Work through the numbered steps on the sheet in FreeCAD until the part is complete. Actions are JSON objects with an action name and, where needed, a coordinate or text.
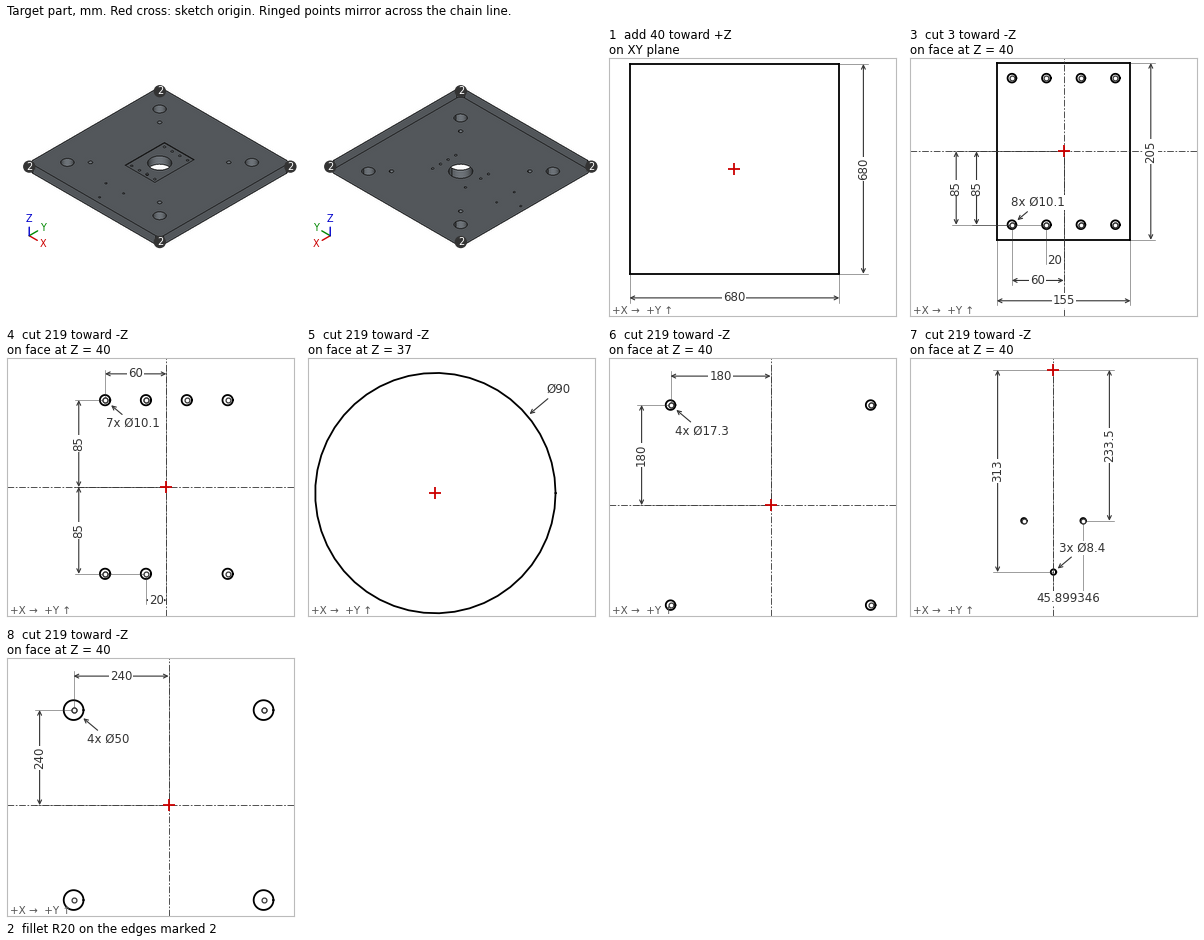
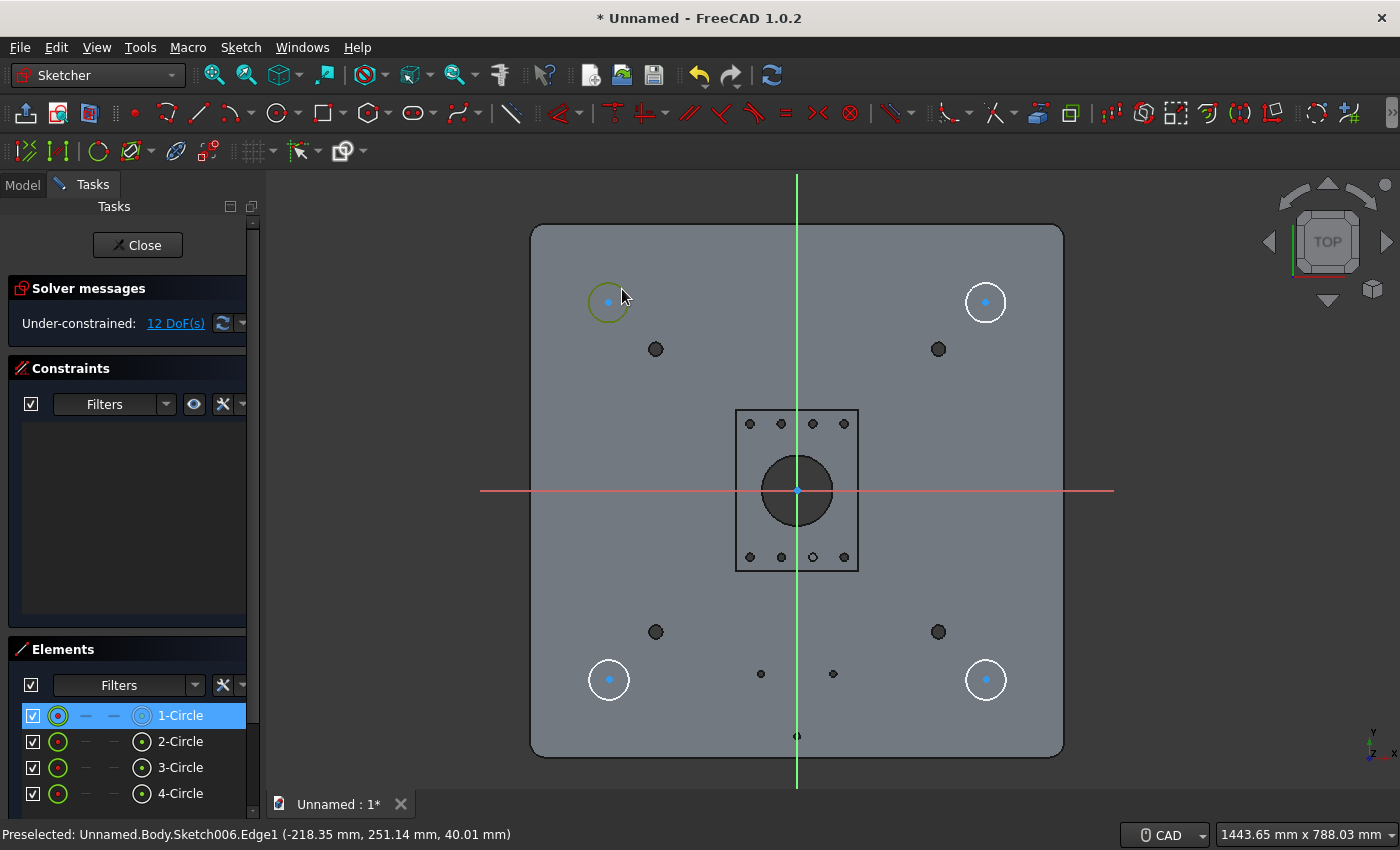
{"action": "left_click", "coordinate": [1000, 289]}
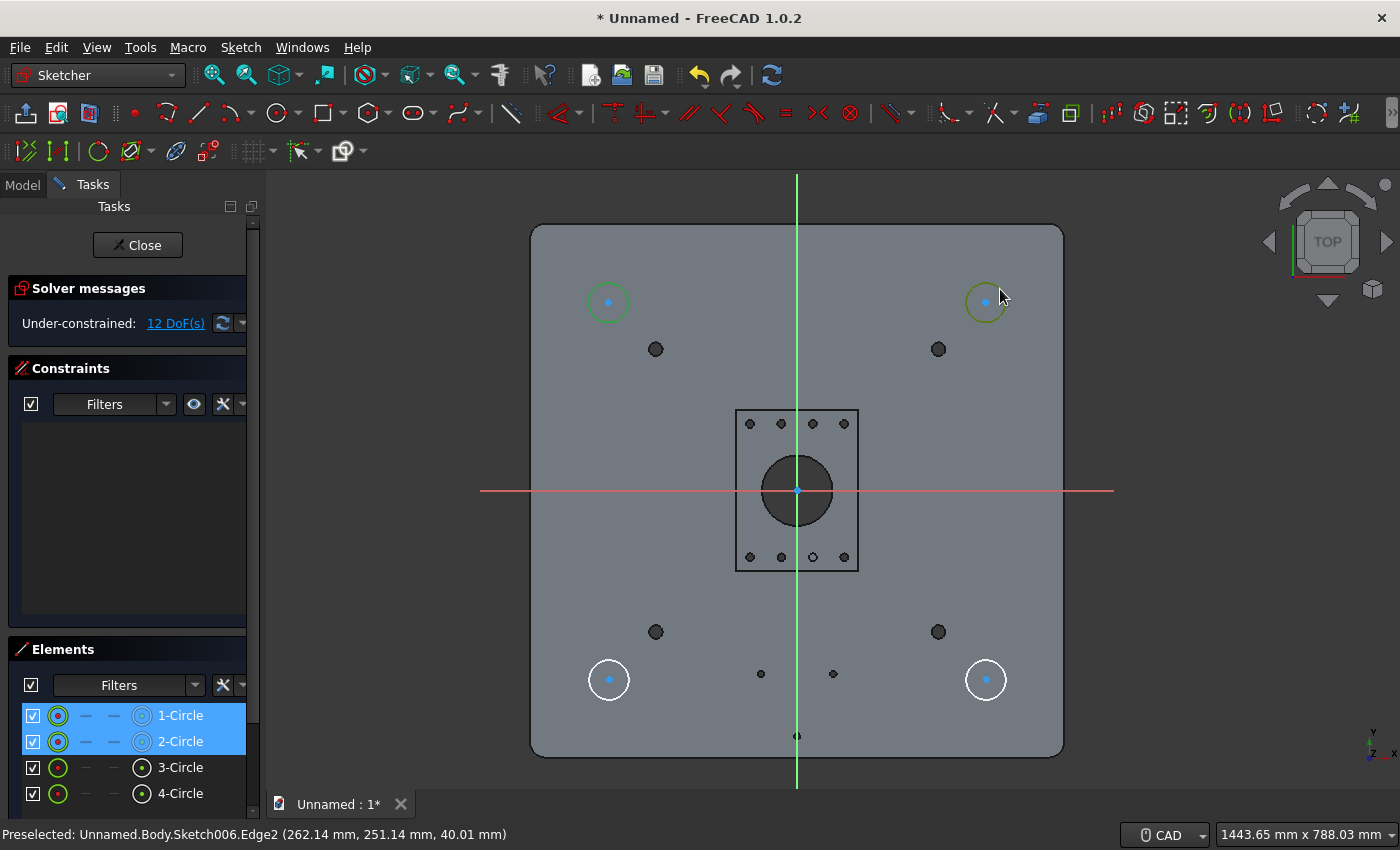
{"action": "left_click", "coordinate": [1000, 666]}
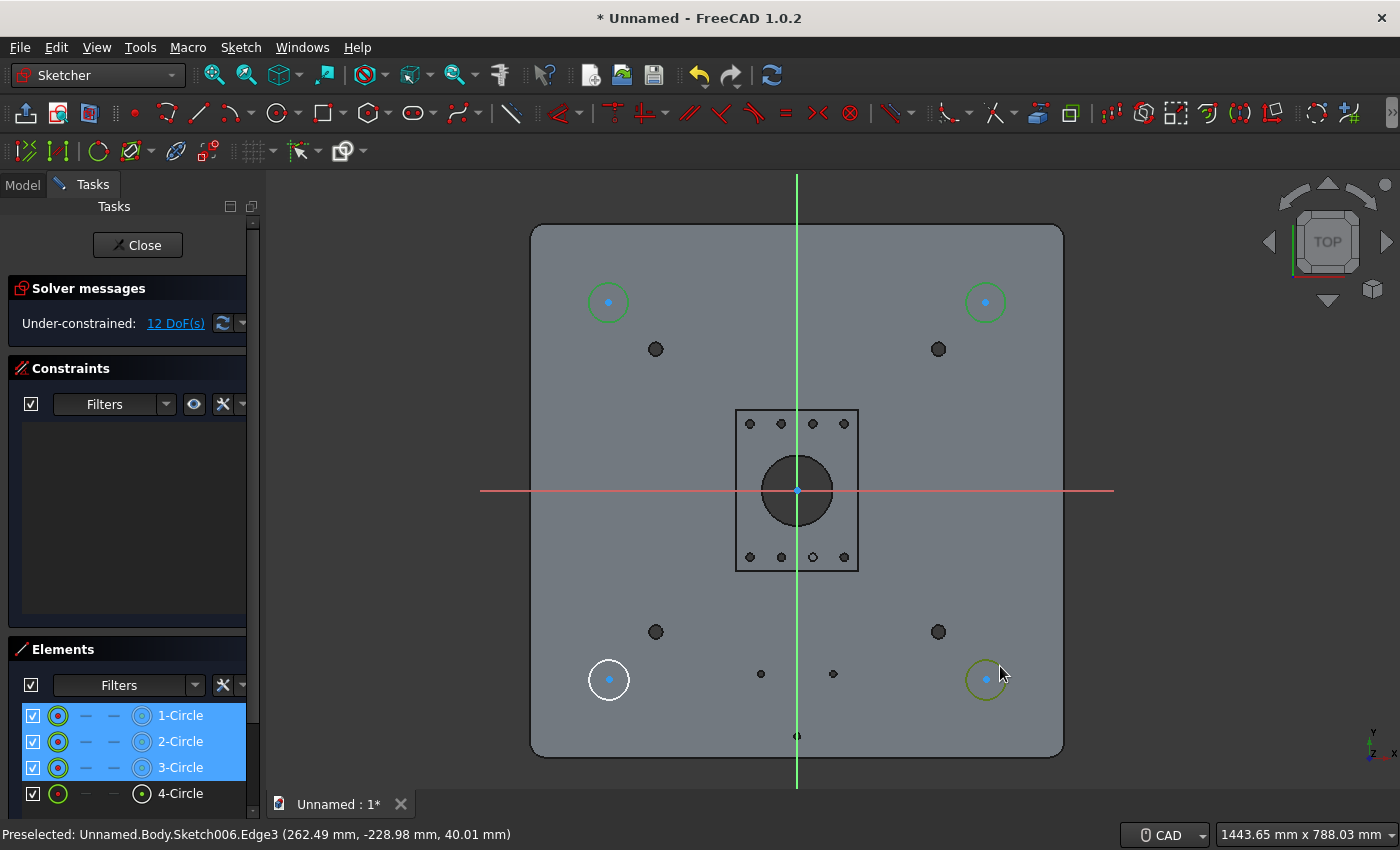
{"action": "left_click", "coordinate": [623, 666]}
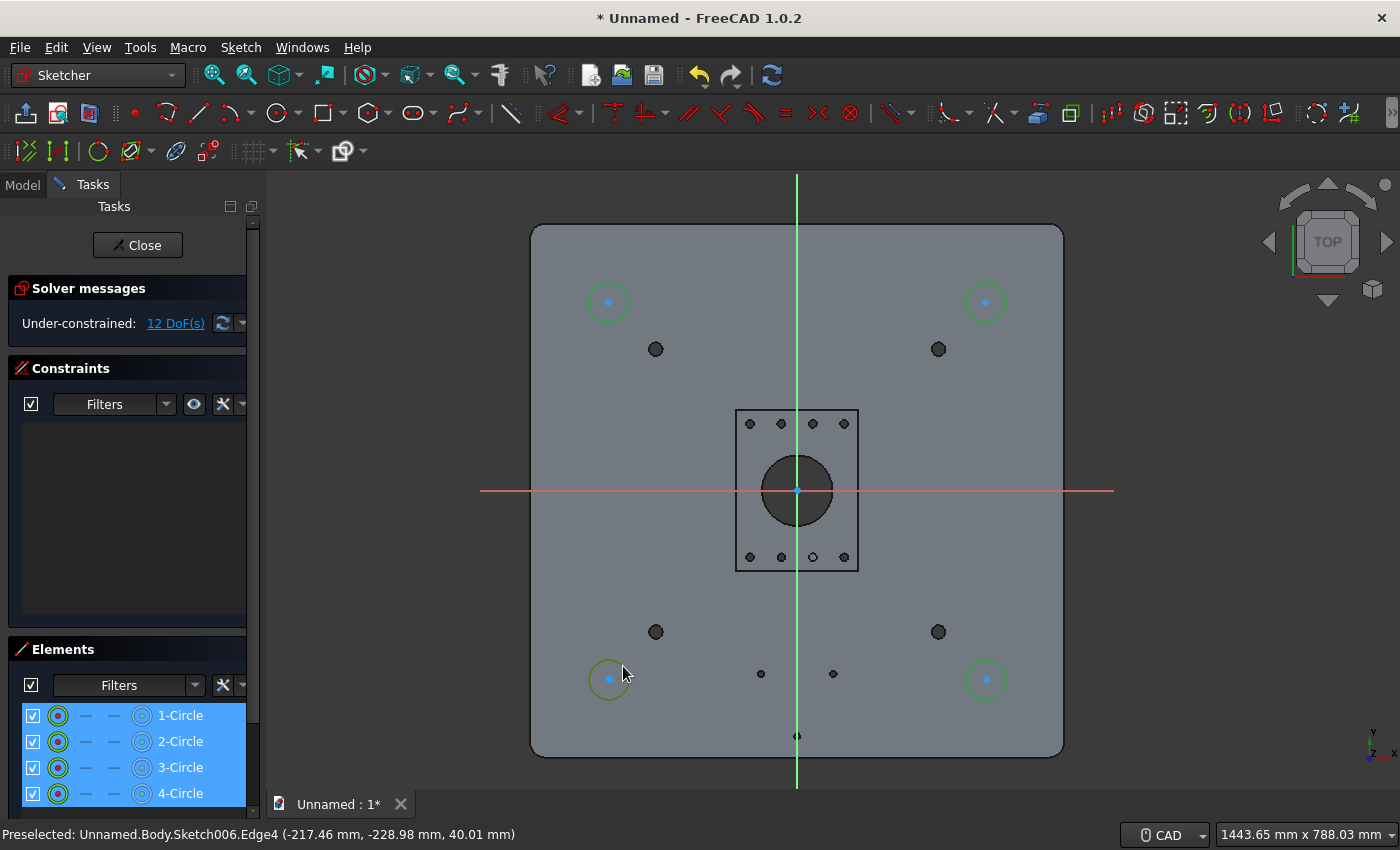
{"action": "left_click", "coordinate": [786, 114]}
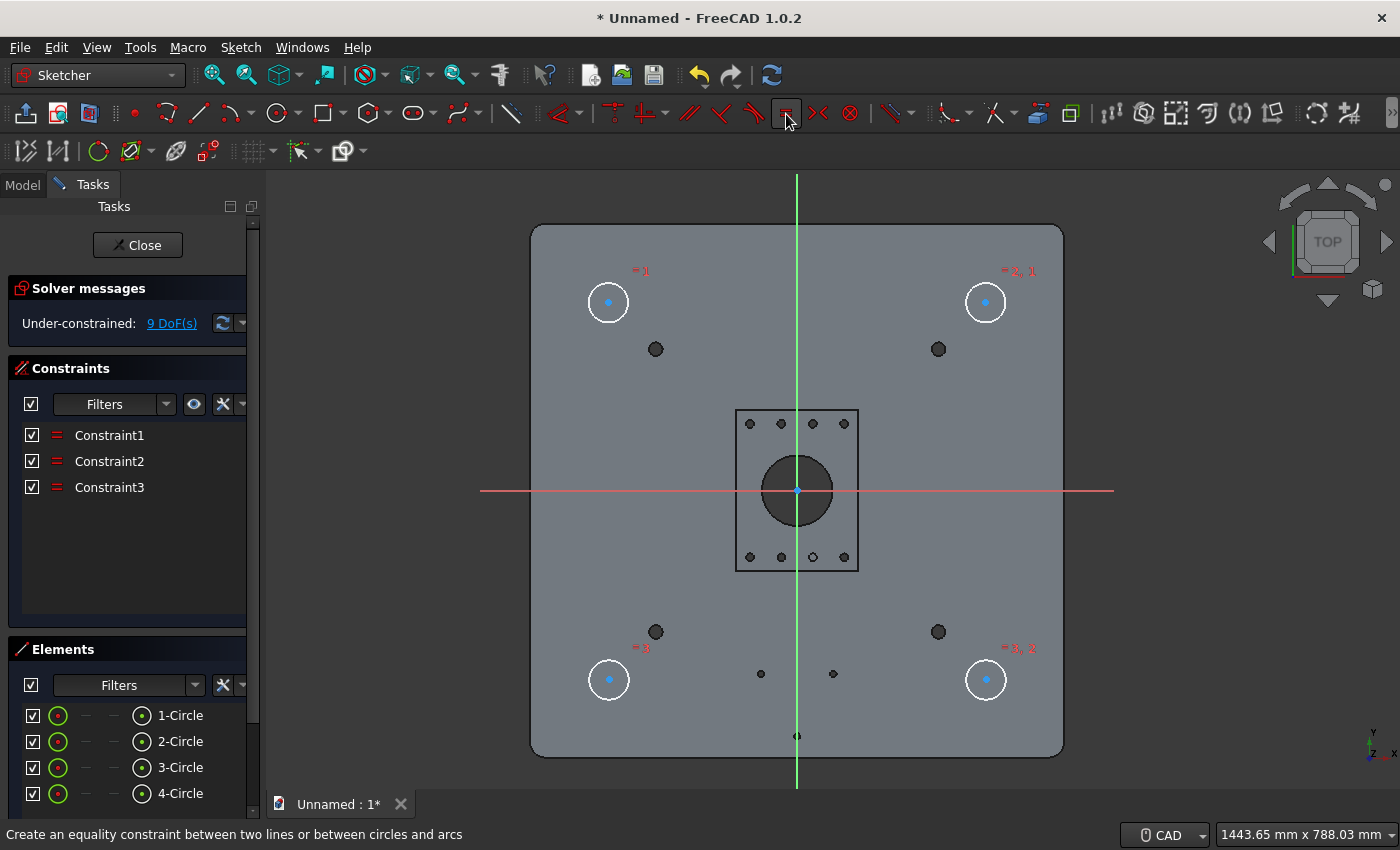
{"action": "left_click", "coordinate": [608, 303]}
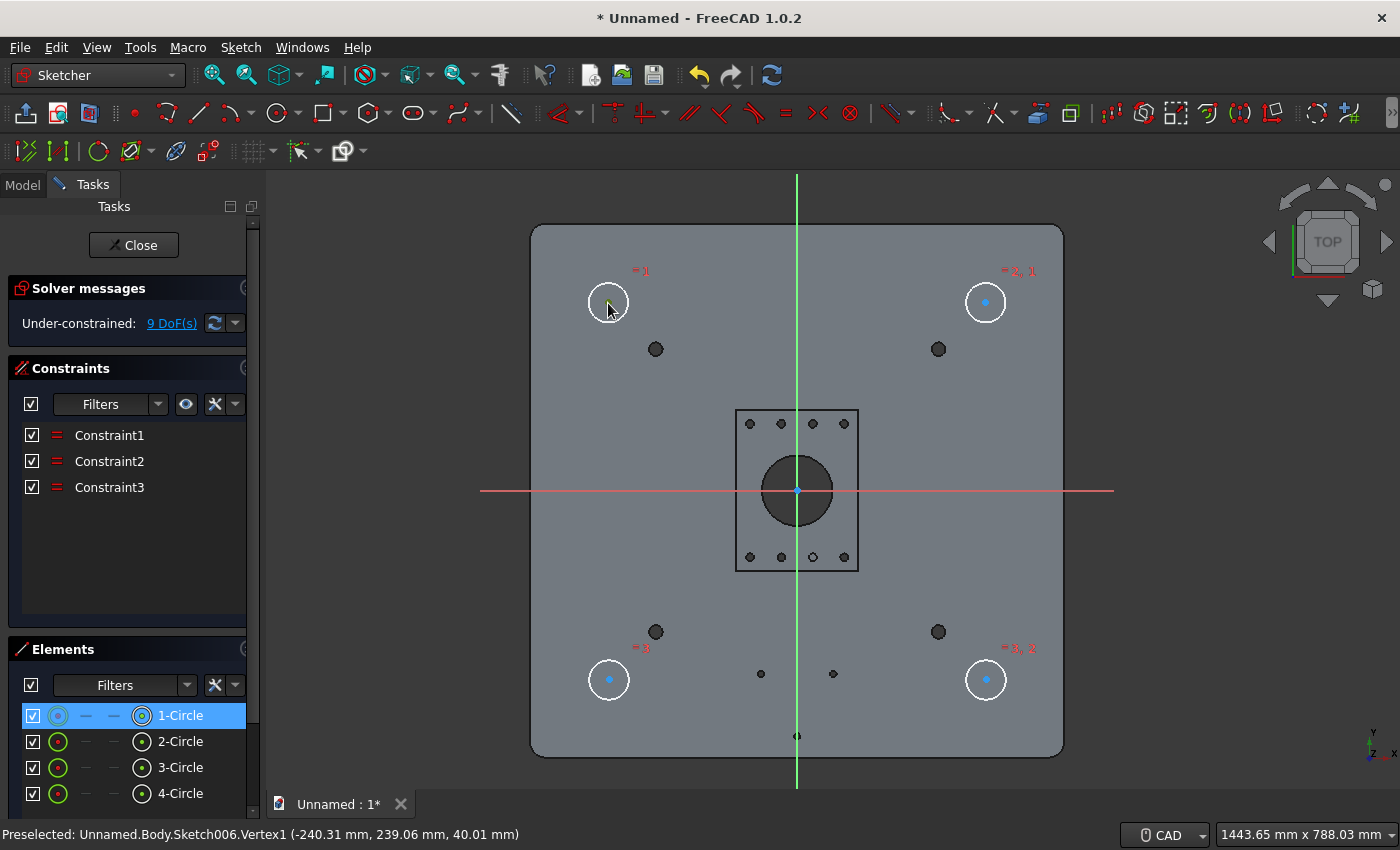
{"action": "left_click", "coordinate": [986, 303]}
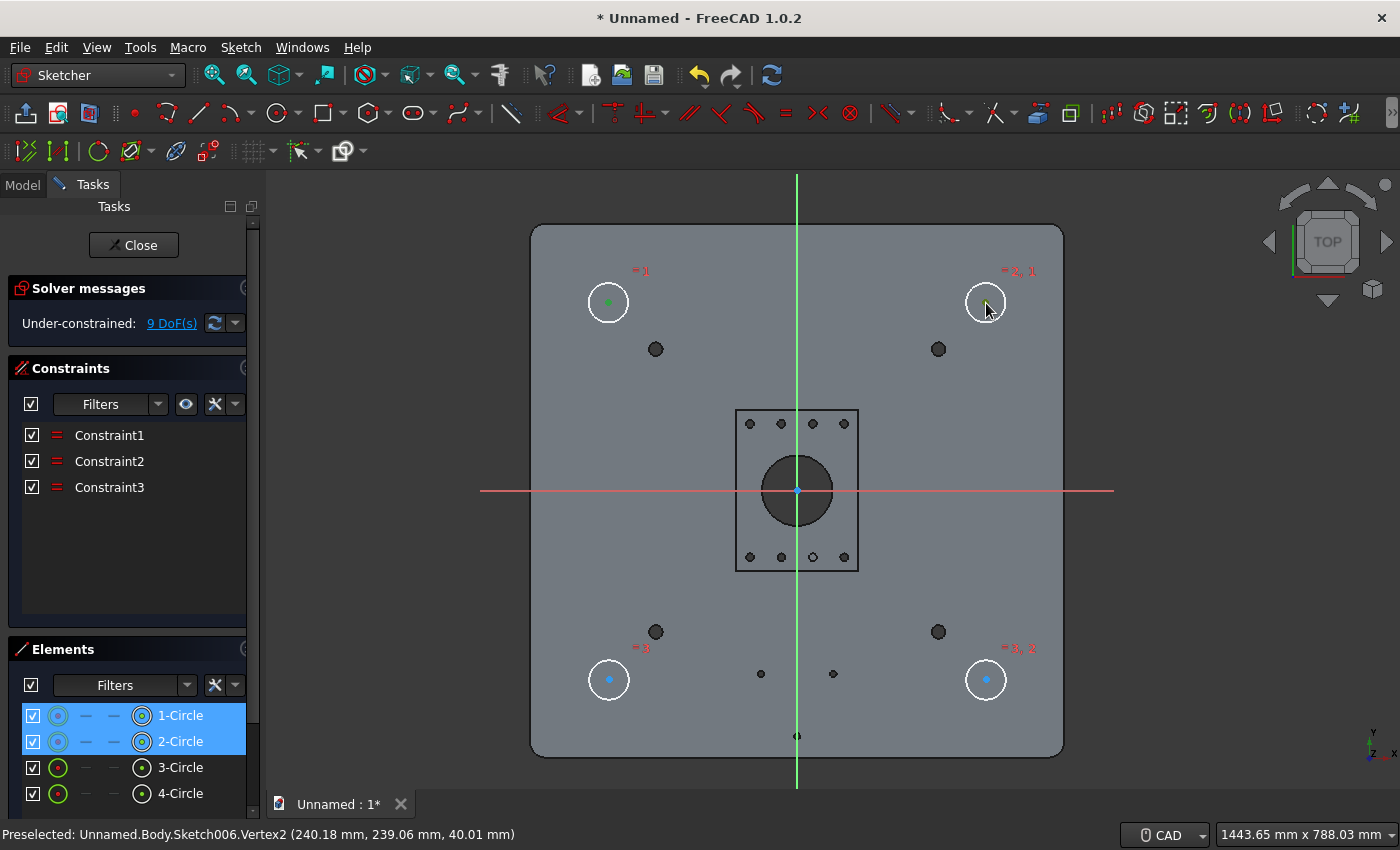
{"action": "left_click", "coordinate": [797, 721]}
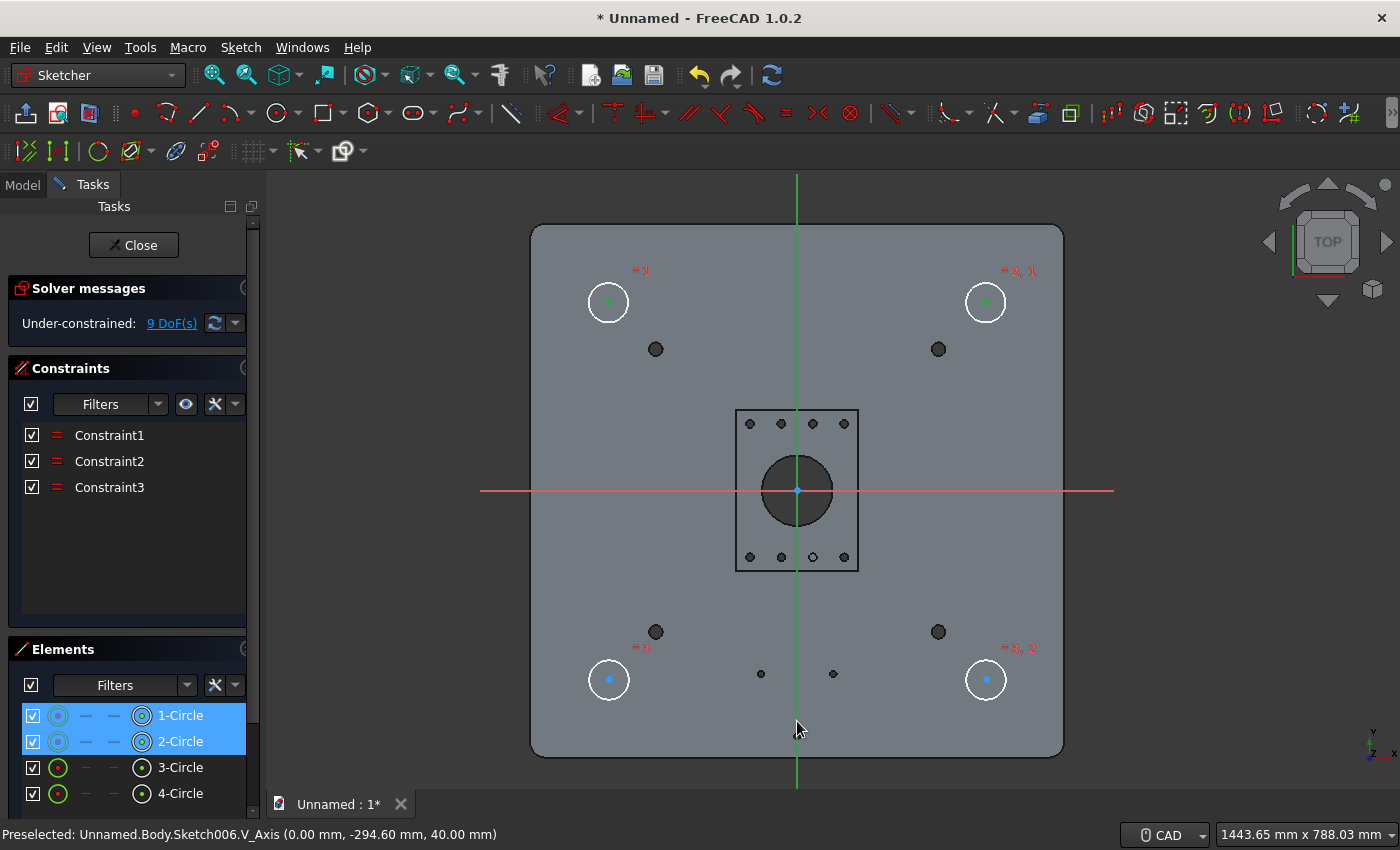
{"action": "left_click", "coordinate": [818, 114]}